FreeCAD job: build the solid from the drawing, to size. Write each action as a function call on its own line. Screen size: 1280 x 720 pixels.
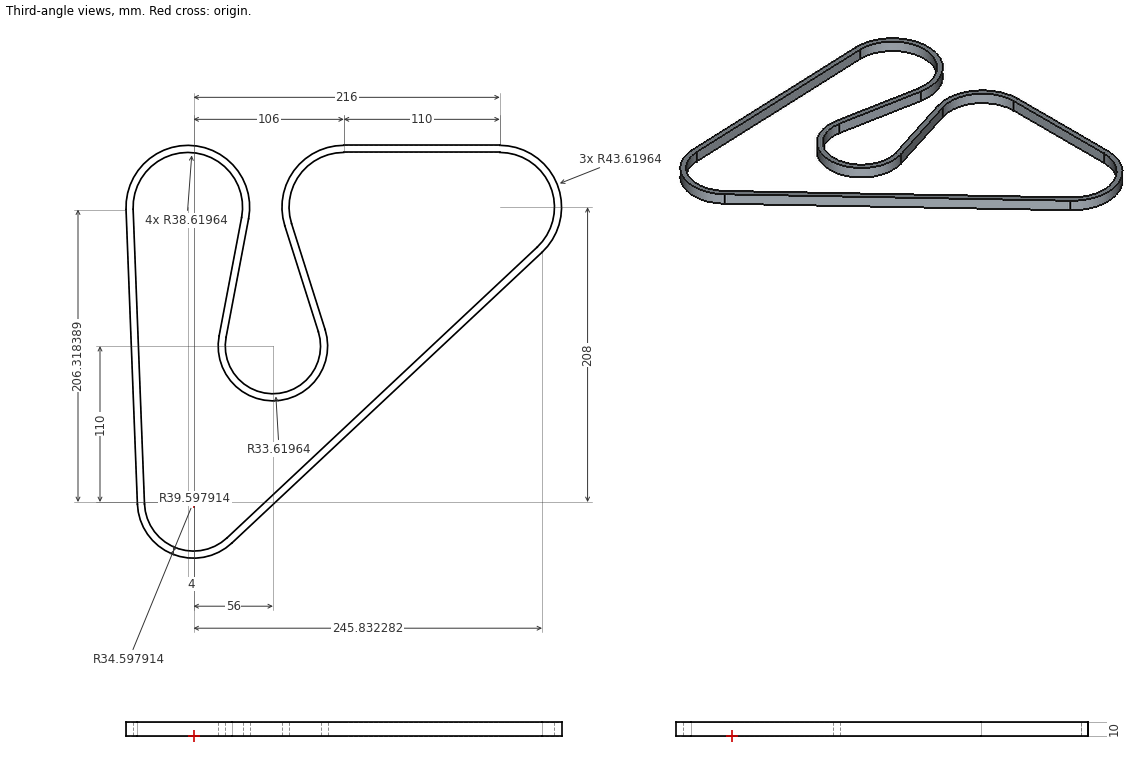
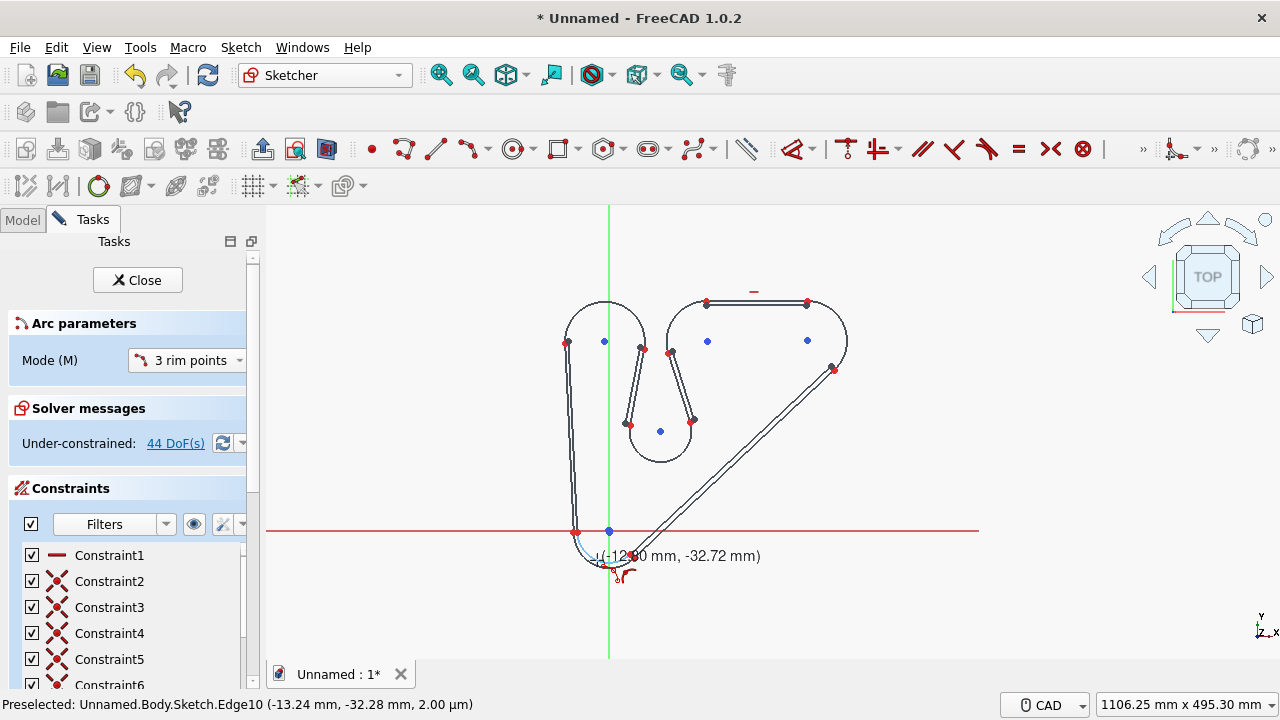
scroll(570, 342, up, 7)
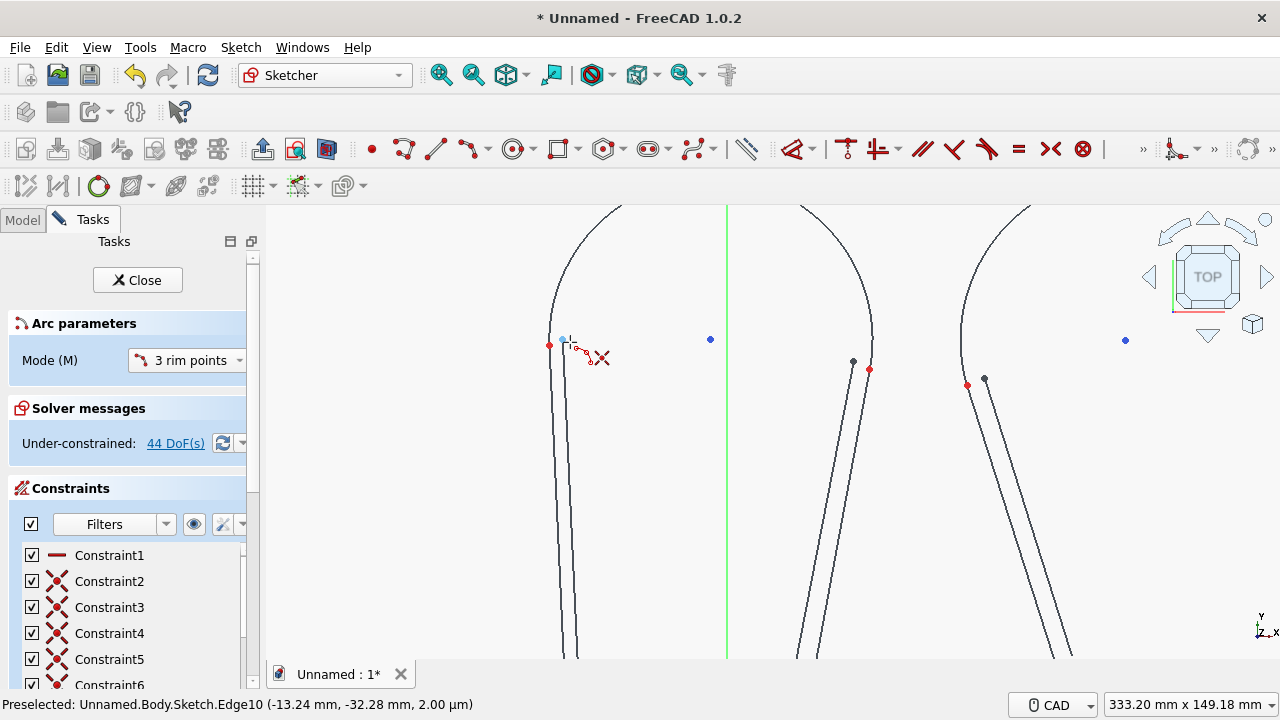
click(563, 340)
click(854, 362)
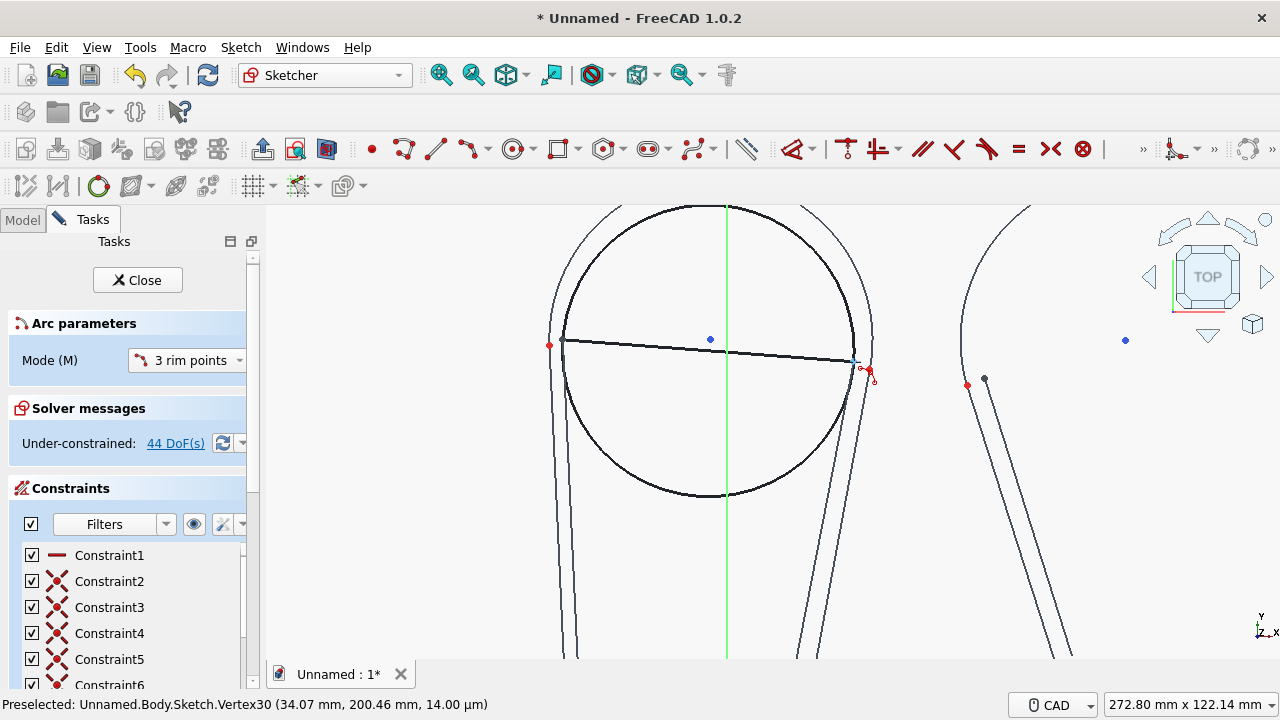
scroll(570, 342, down, 7)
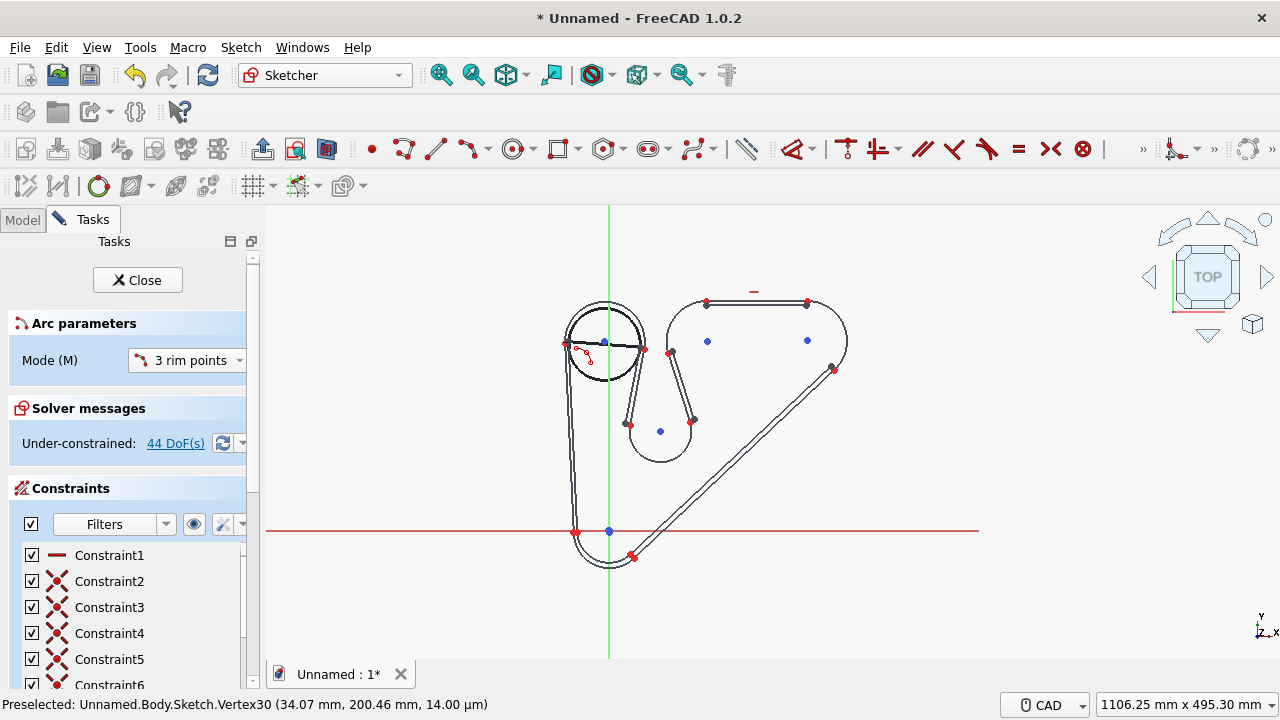
scroll(619, 308, up, 7)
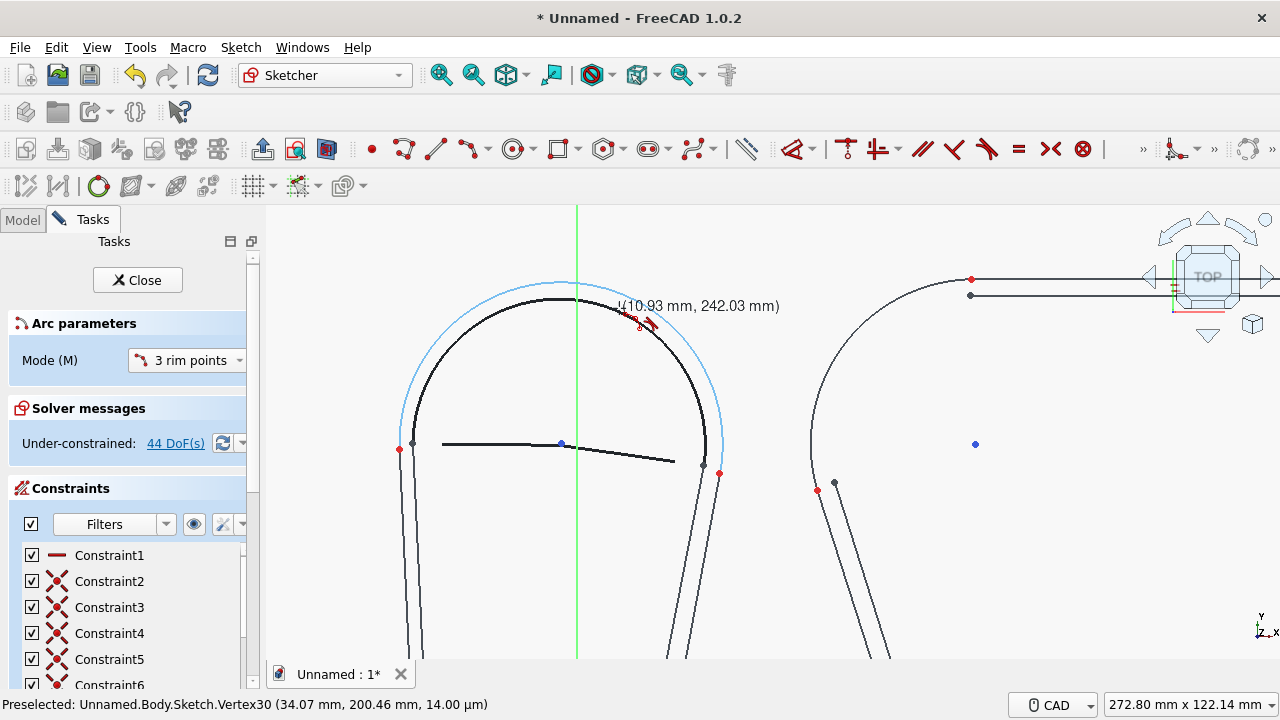
click(620, 306)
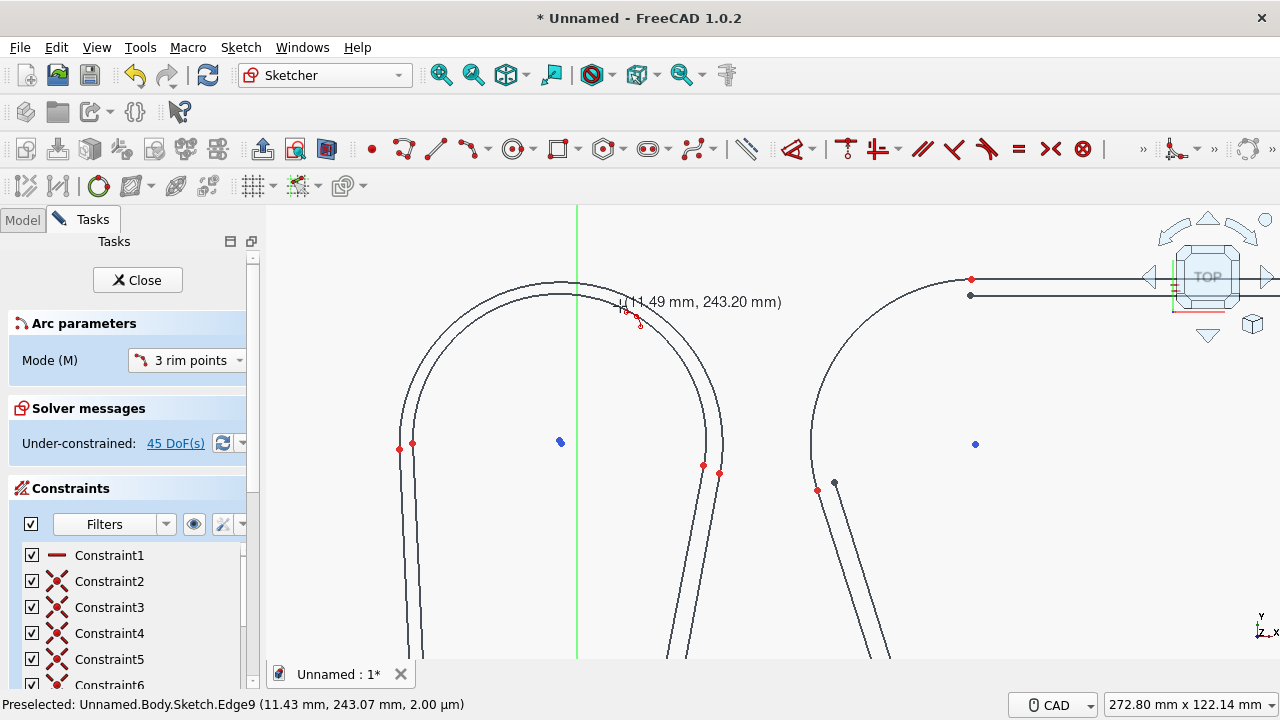
scroll(619, 308, down, 7)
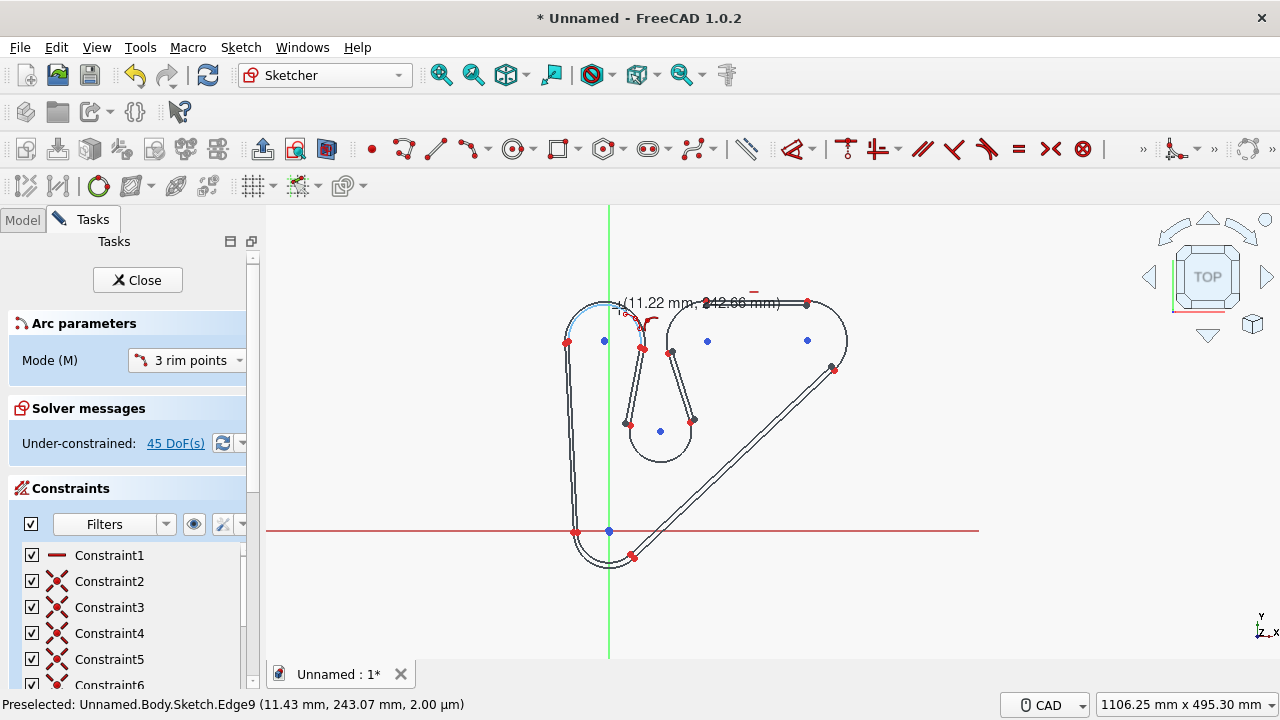
scroll(626, 423, up, 7)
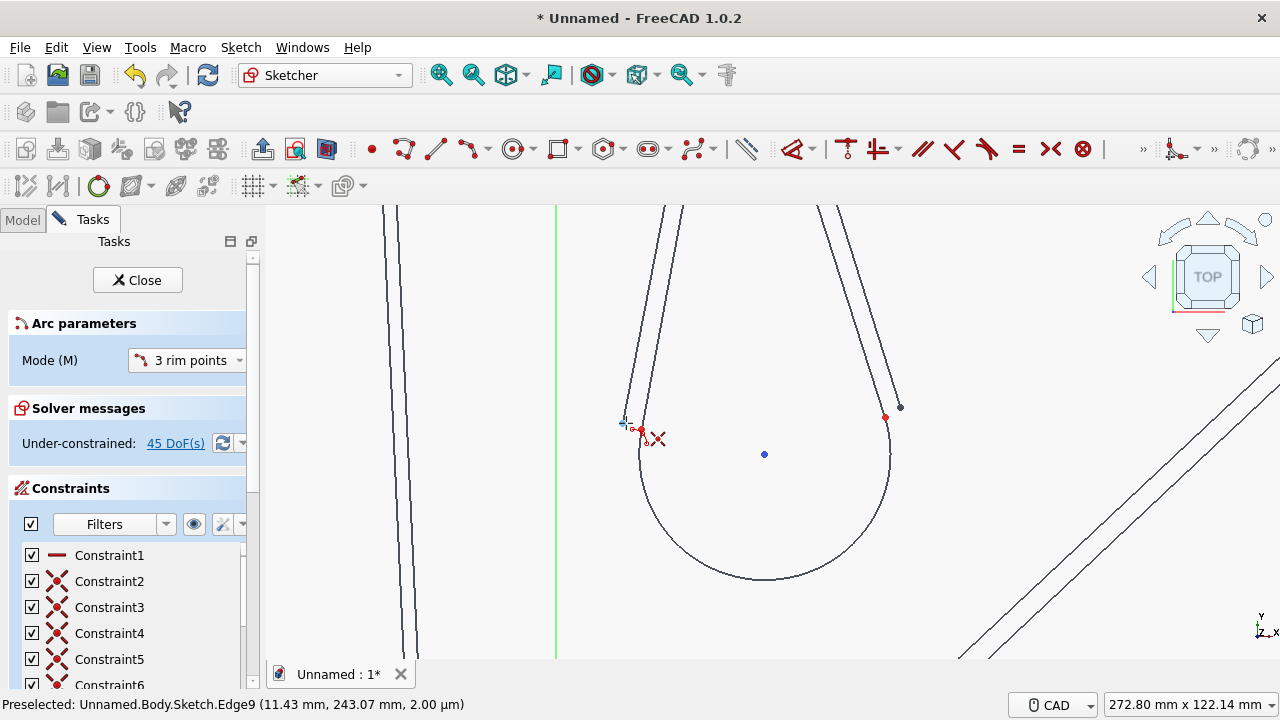
click(623, 424)
click(901, 408)
click(823, 581)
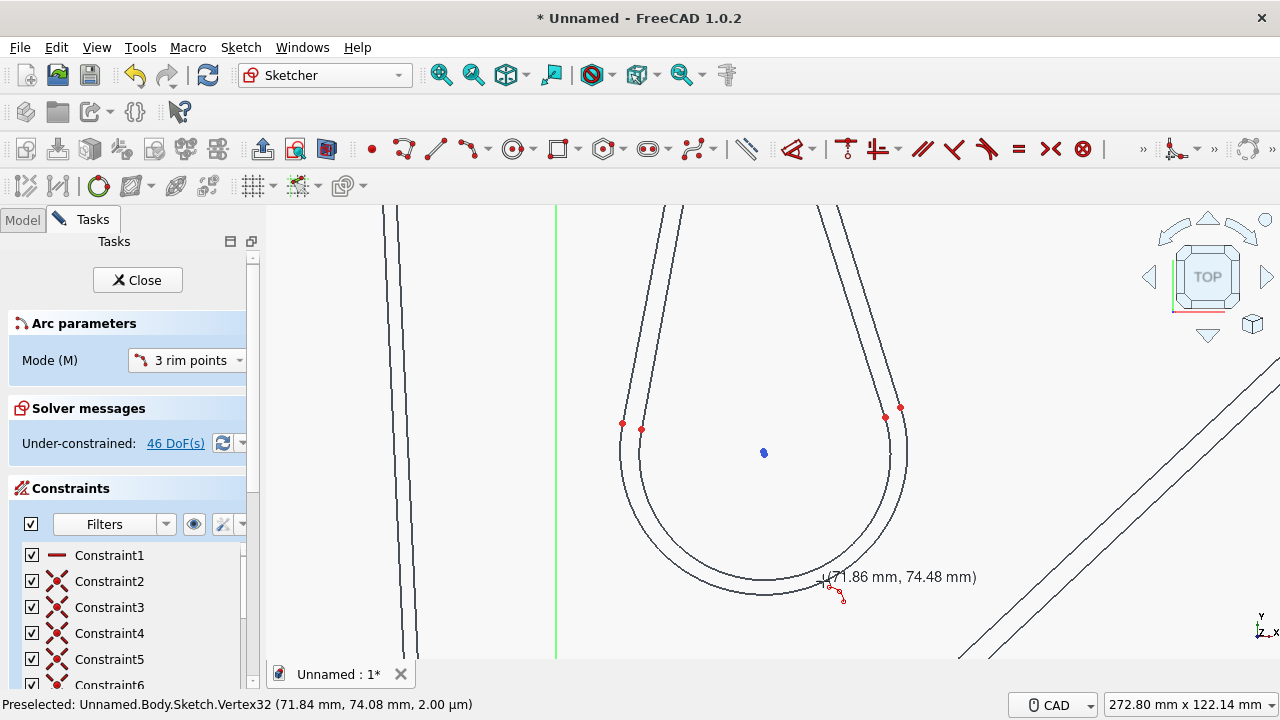
scroll(626, 423, down, 7)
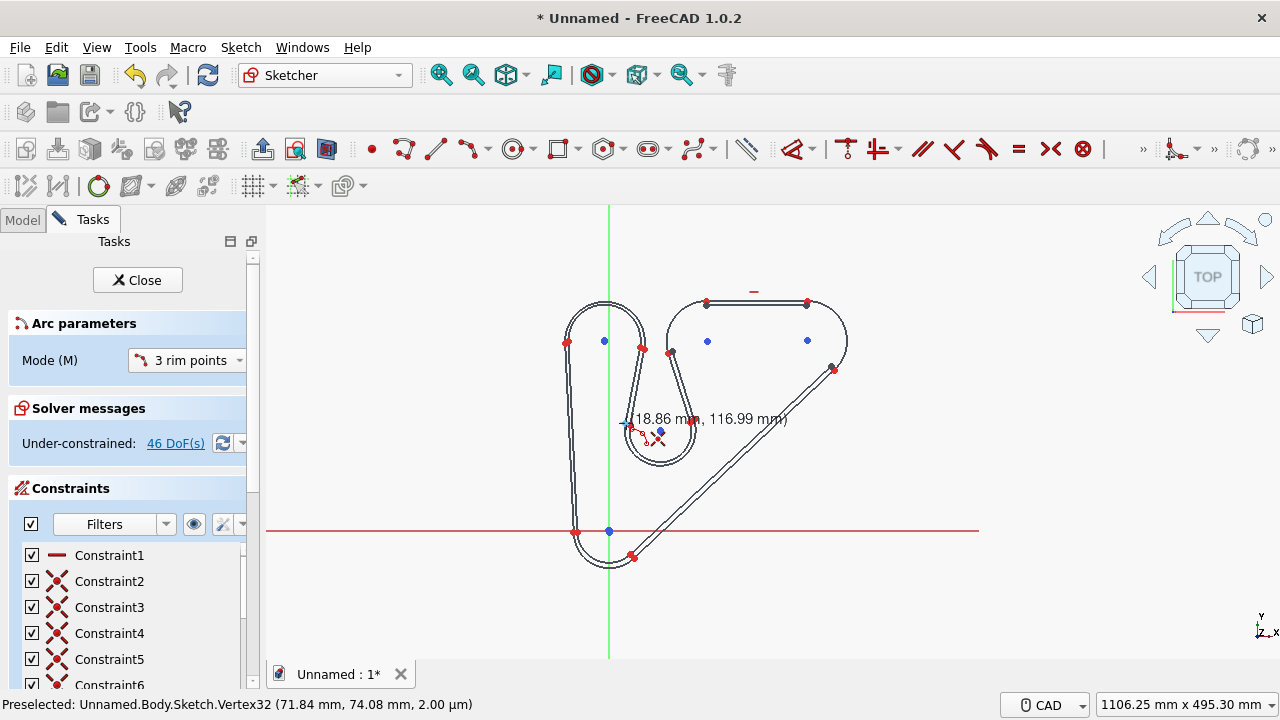
scroll(672, 351, up, 7)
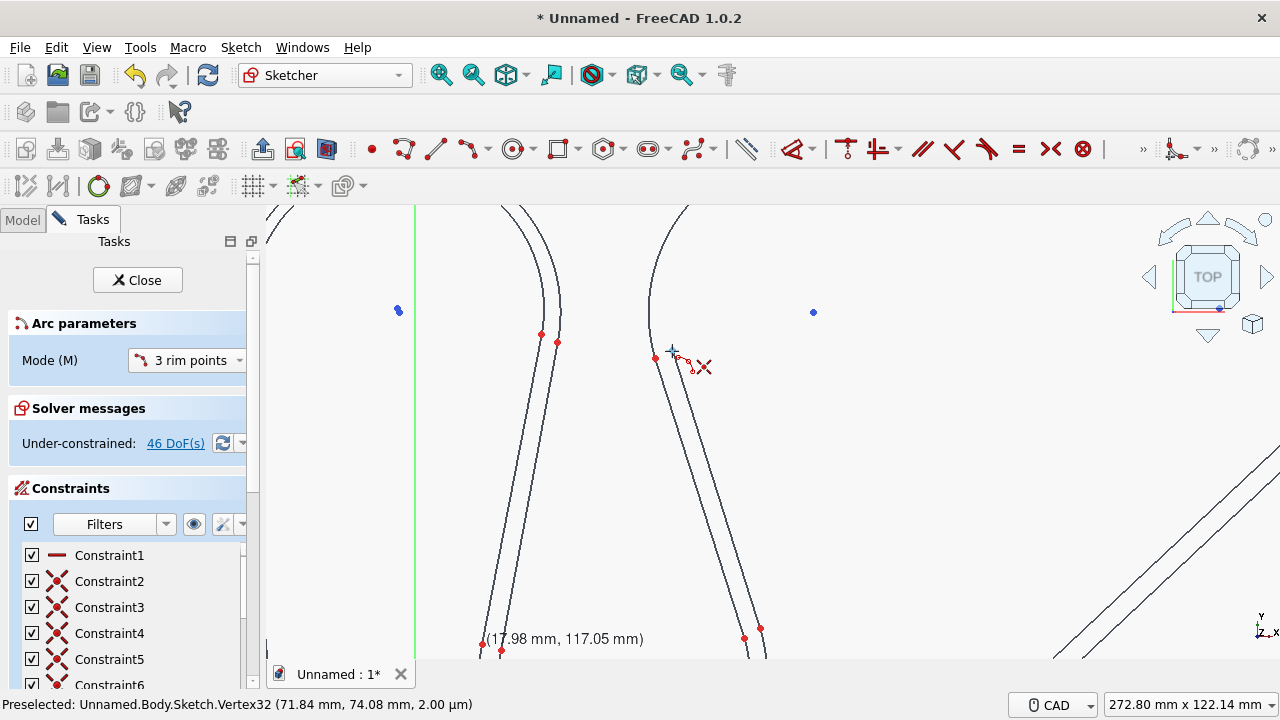
click(673, 351)